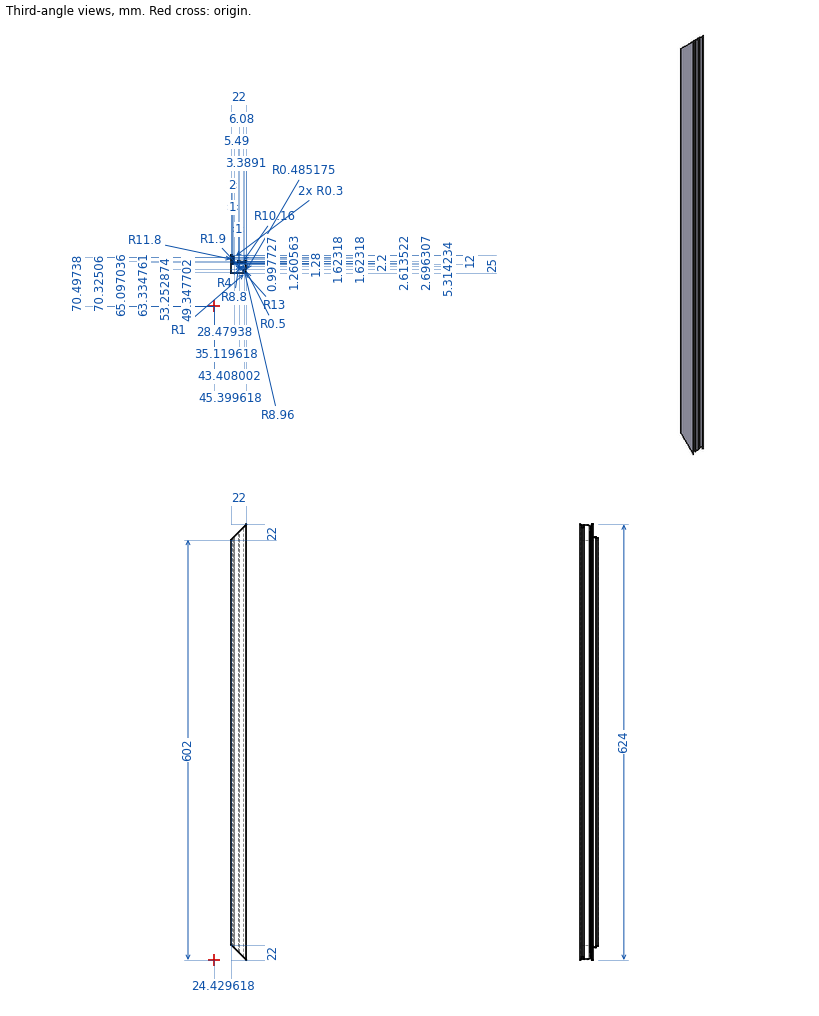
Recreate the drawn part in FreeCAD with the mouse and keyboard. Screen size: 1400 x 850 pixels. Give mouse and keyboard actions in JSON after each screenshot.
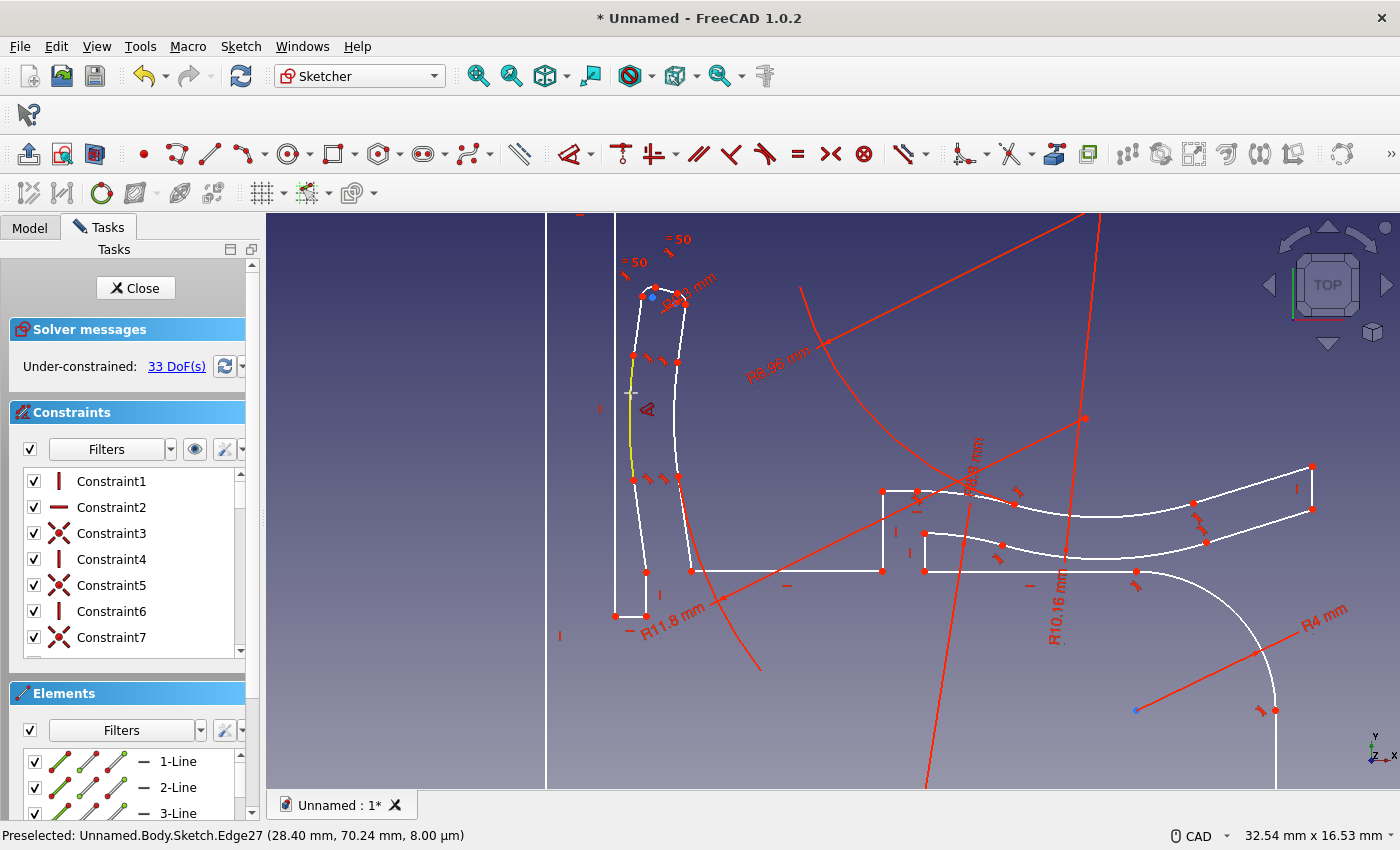
{"action": "left_click", "coordinate": [630, 393]}
{"action": "left_click", "coordinate": [598, 391]}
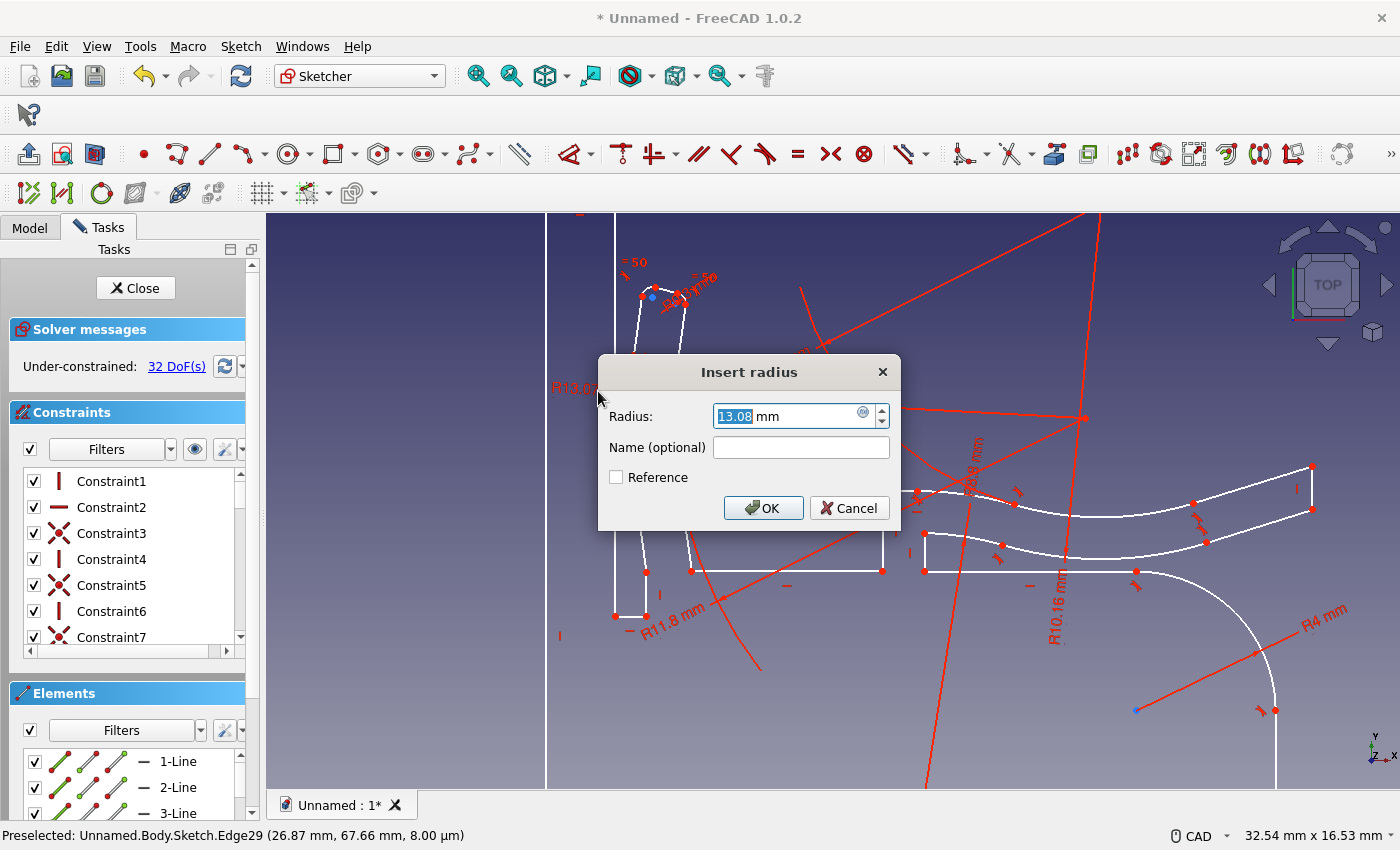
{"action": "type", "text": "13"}
{"action": "key", "text": "Return"}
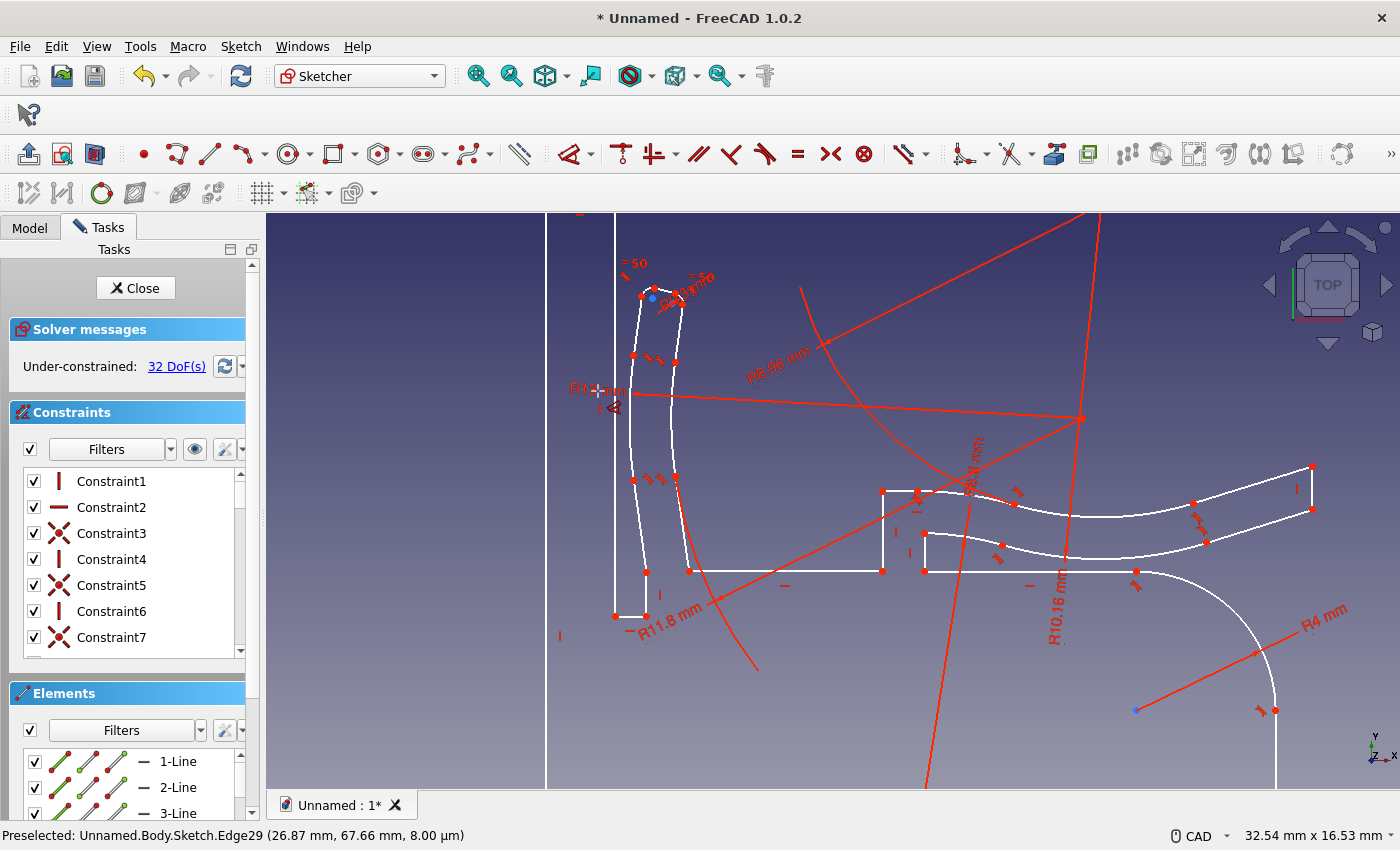
{"action": "scroll", "coordinate": [631, 393], "scroll_direction": "down", "scroll_amount": 4}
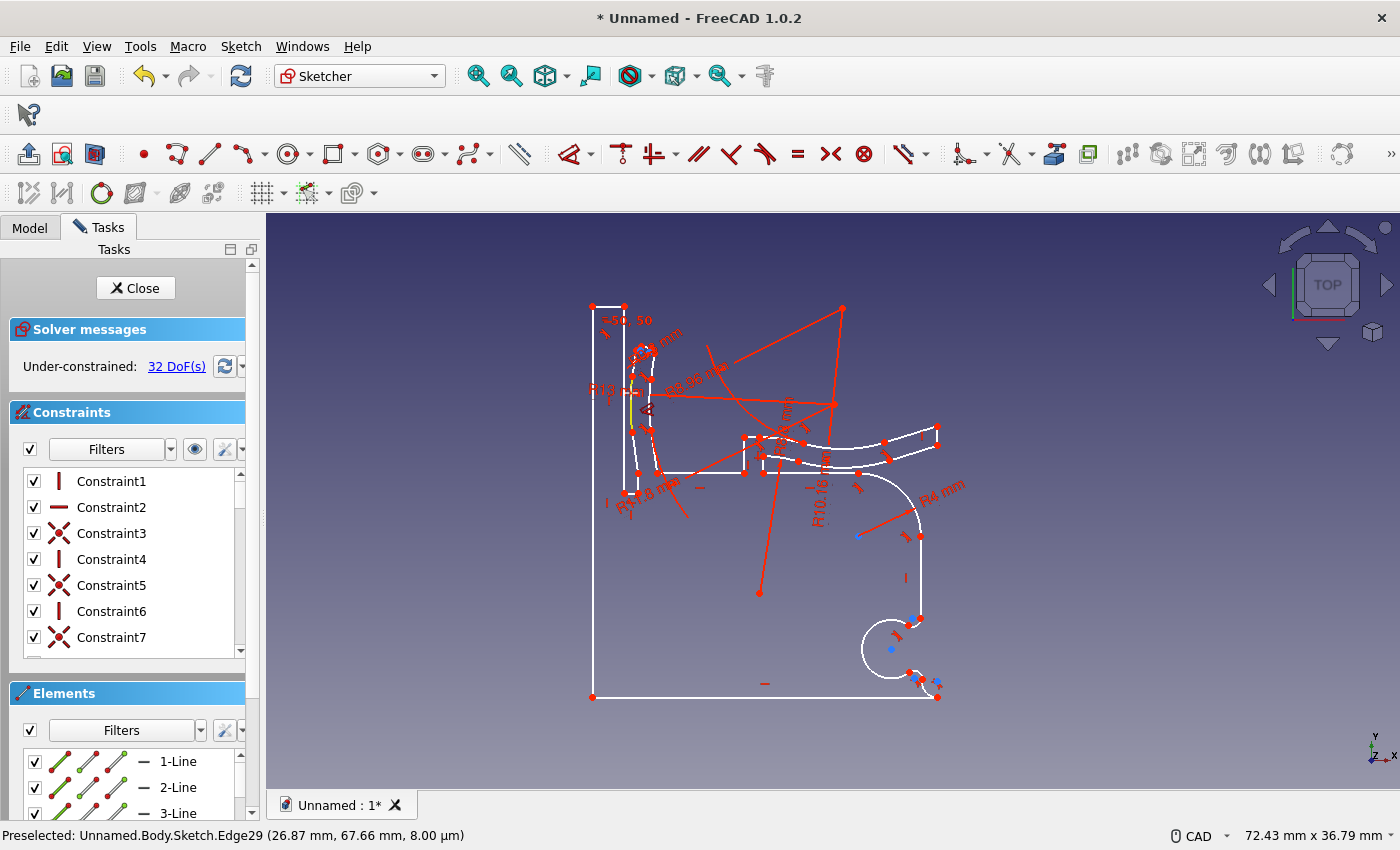
{"action": "scroll", "coordinate": [923, 688], "scroll_direction": "up", "scroll_amount": 5}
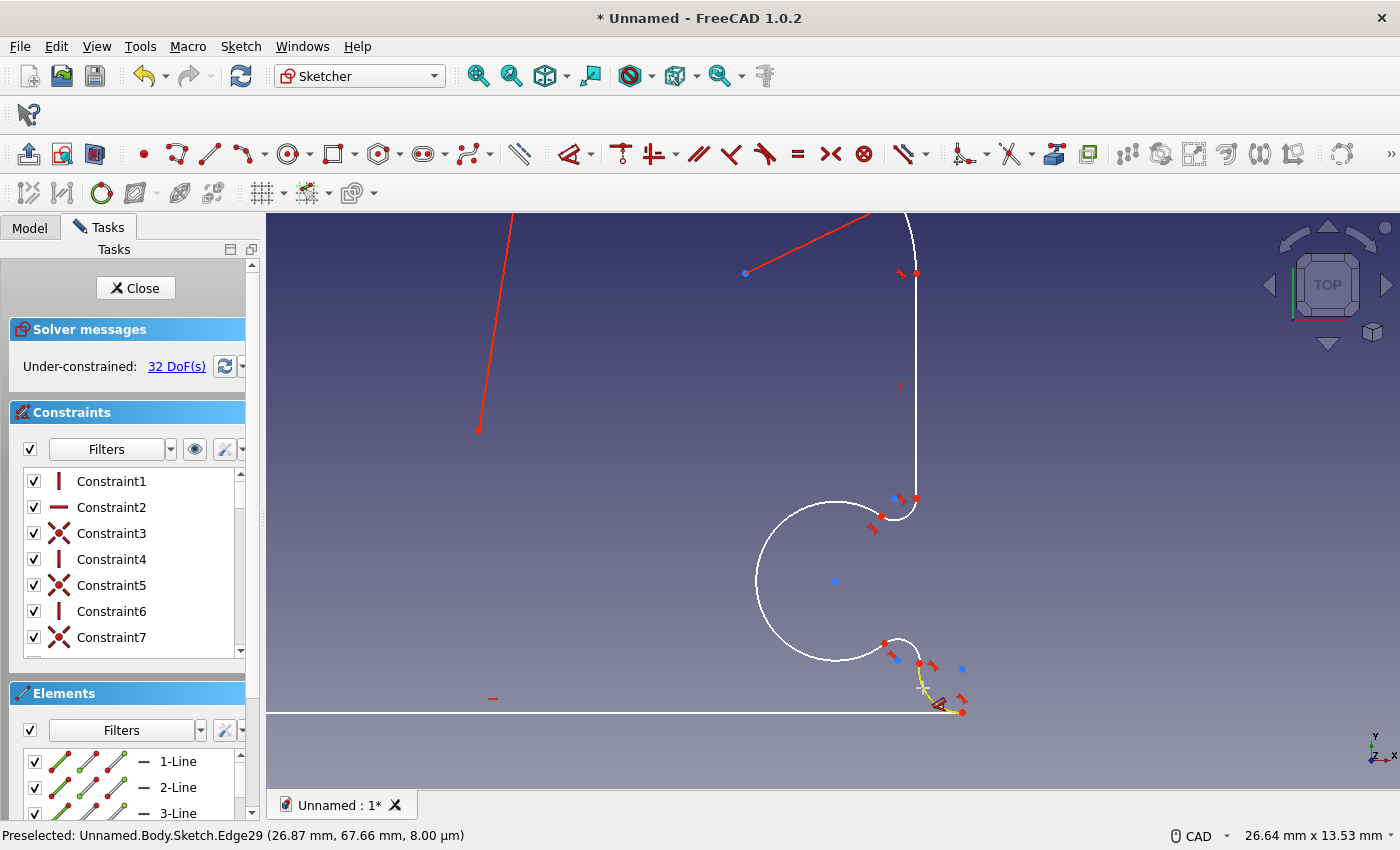
{"action": "left_click", "coordinate": [922, 686]}
{"action": "left_click", "coordinate": [892, 698]}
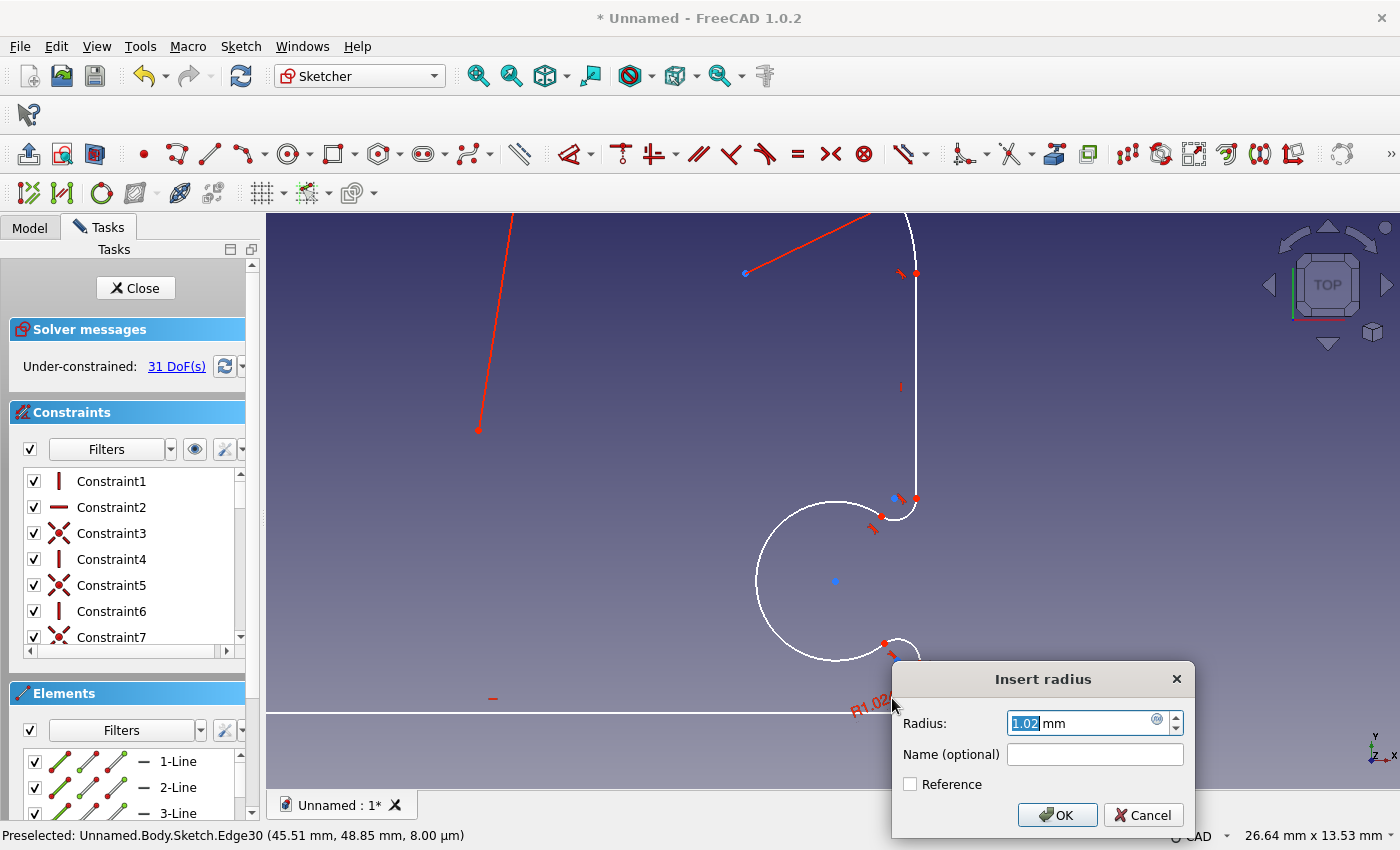
{"action": "type", "text": "1"}
{"action": "key", "text": "Return"}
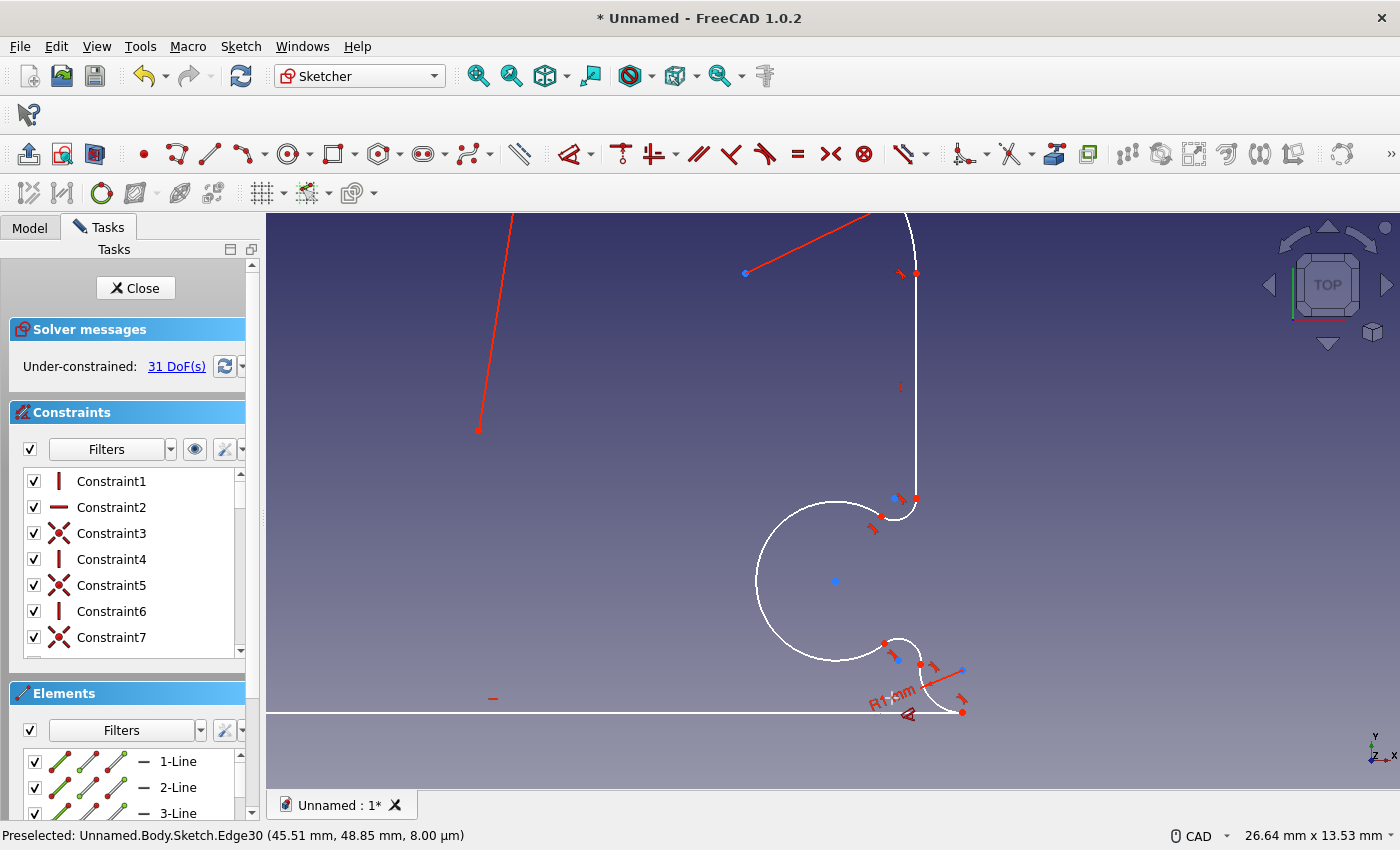
{"action": "scroll", "coordinate": [917, 649], "scroll_direction": "up", "scroll_amount": 4}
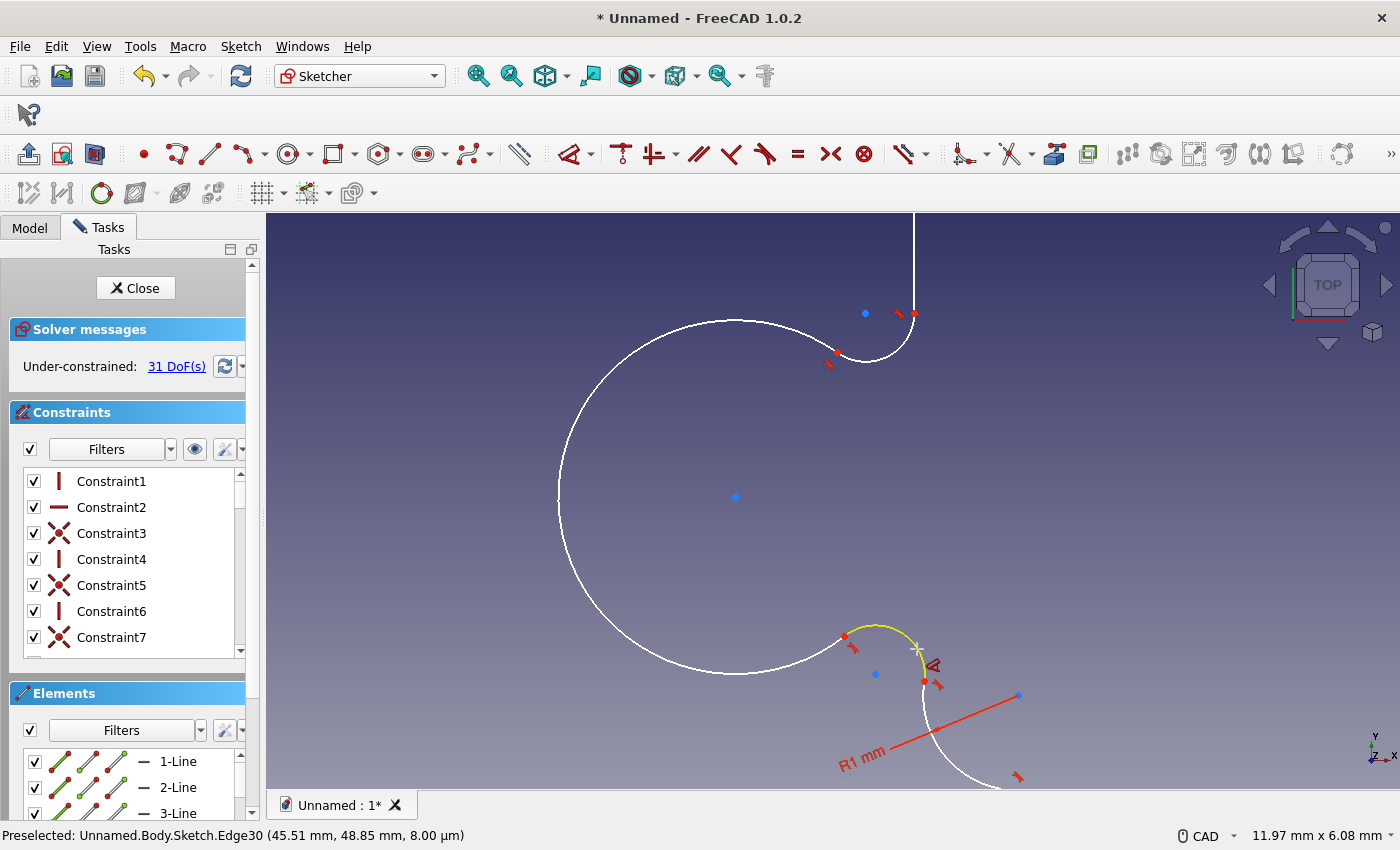
{"action": "left_click", "coordinate": [917, 648]}
{"action": "left_click", "coordinate": [944, 631]}